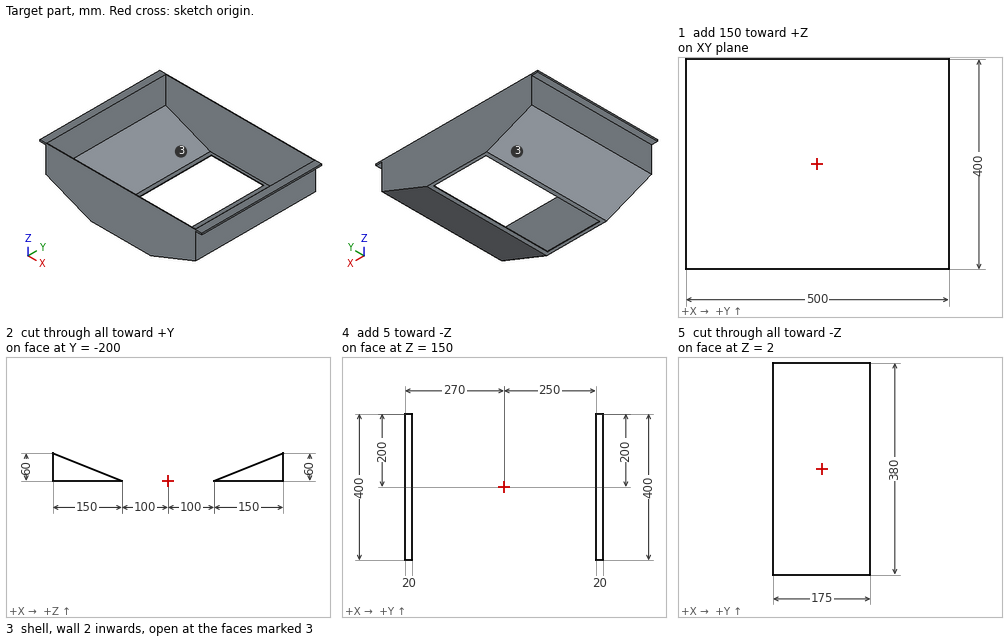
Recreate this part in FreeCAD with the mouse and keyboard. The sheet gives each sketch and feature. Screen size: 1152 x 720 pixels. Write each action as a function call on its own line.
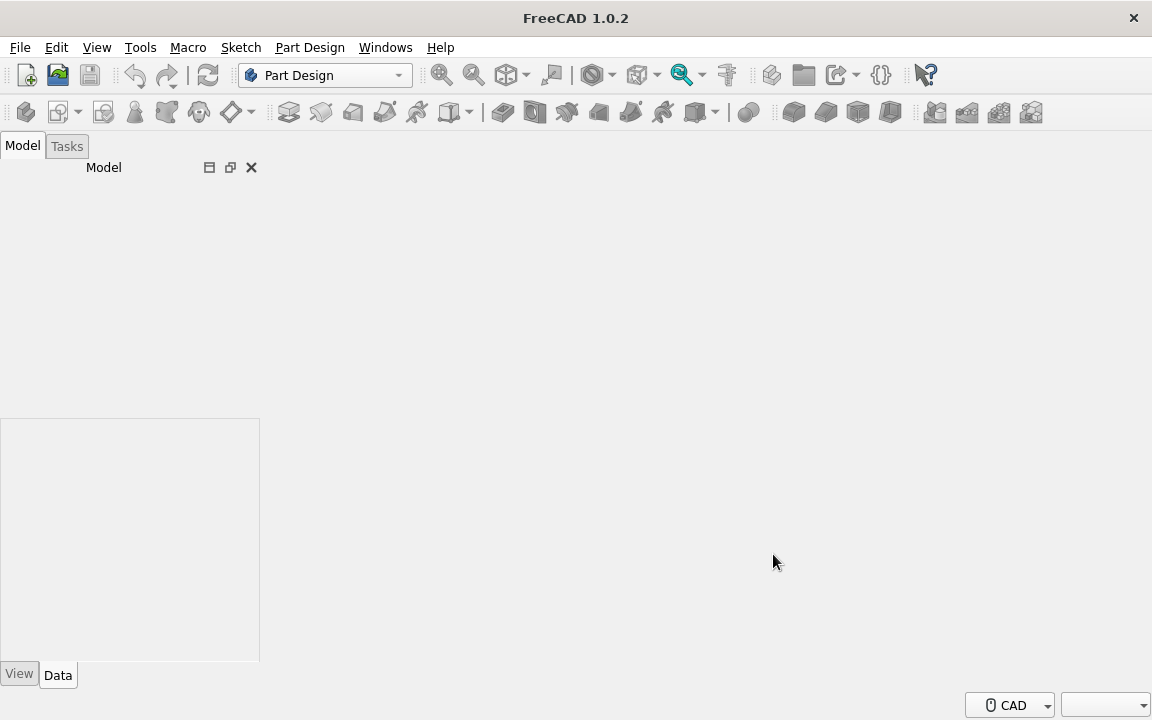
key(ctrl+n)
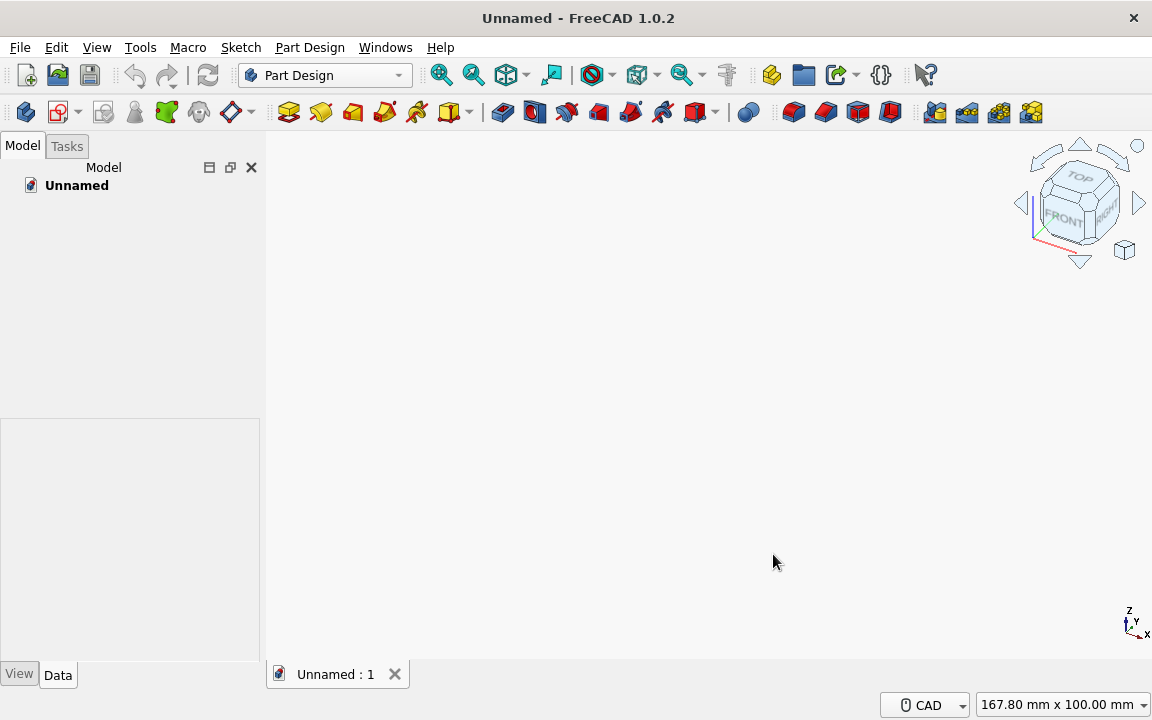
click(58, 112)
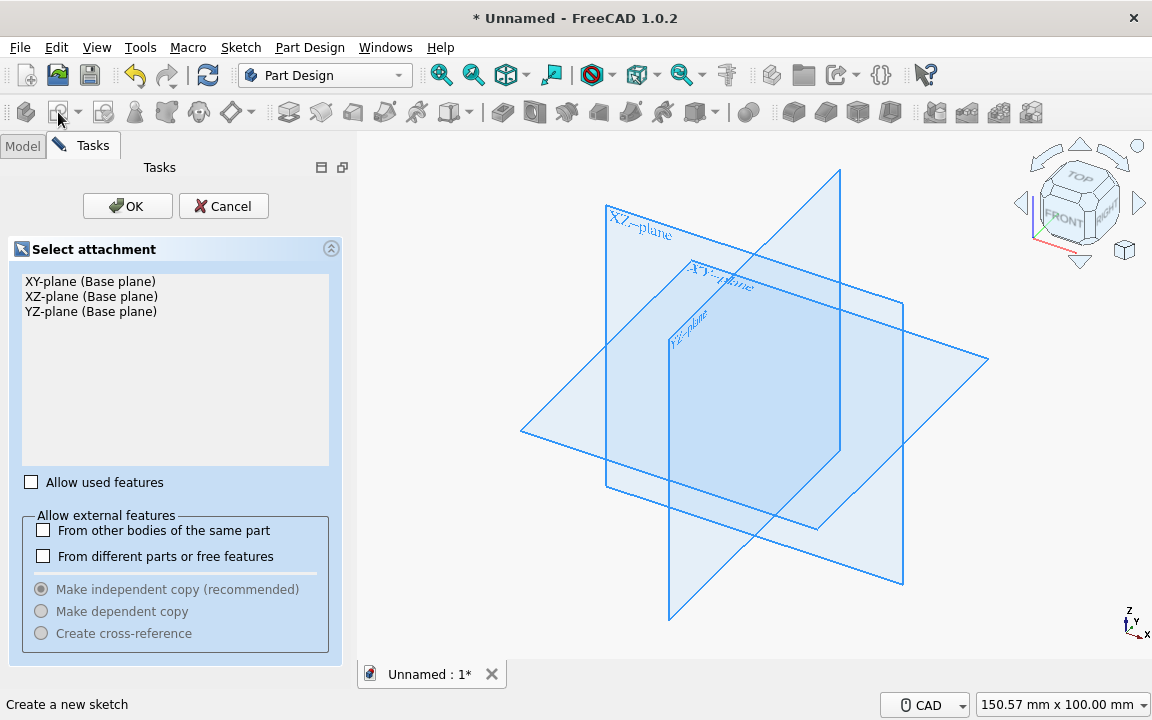
click(82, 282)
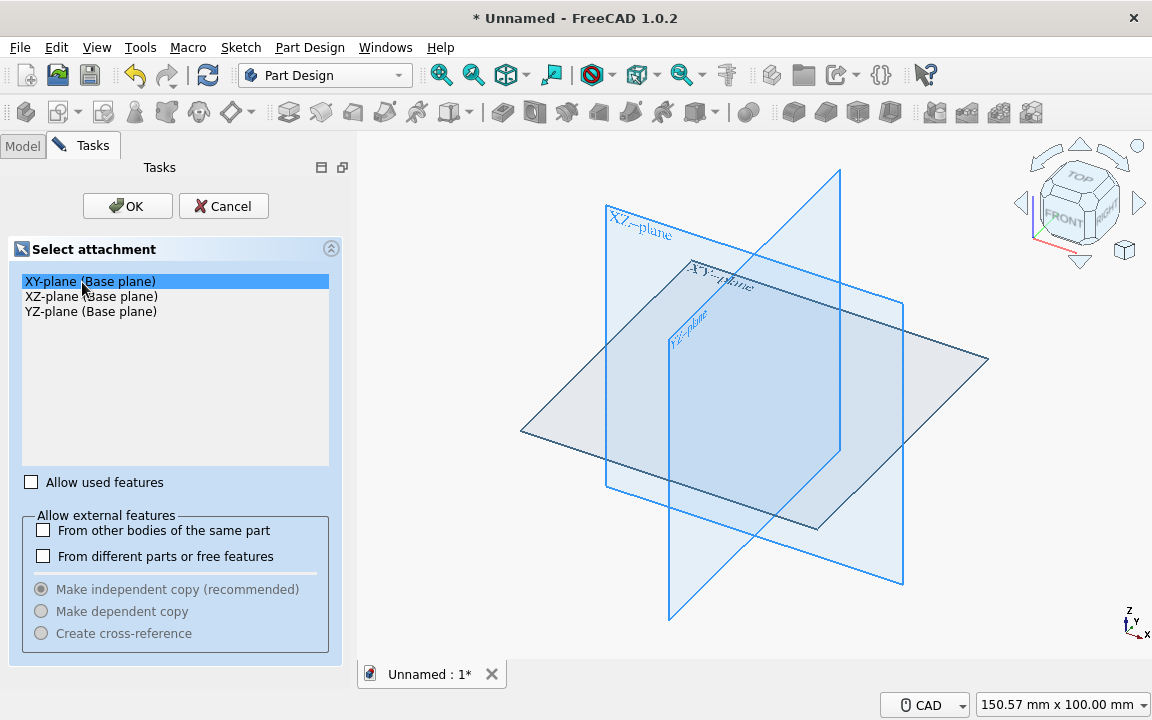
click(128, 206)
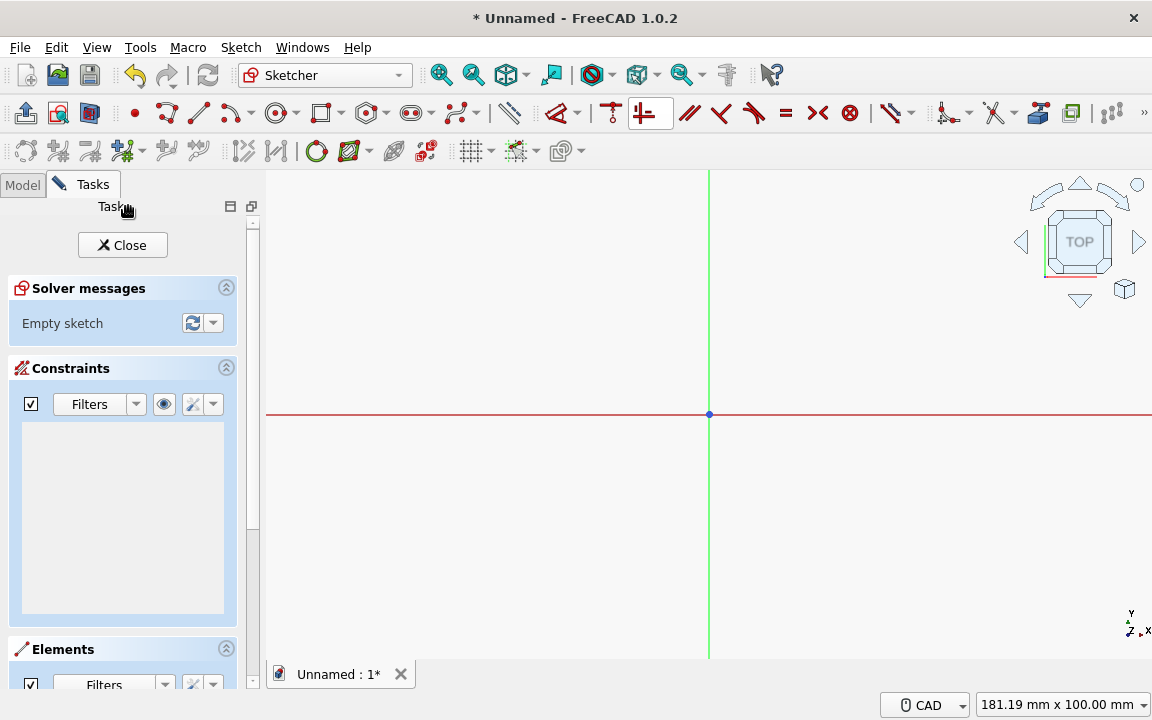
scroll(627, 415, down, 9)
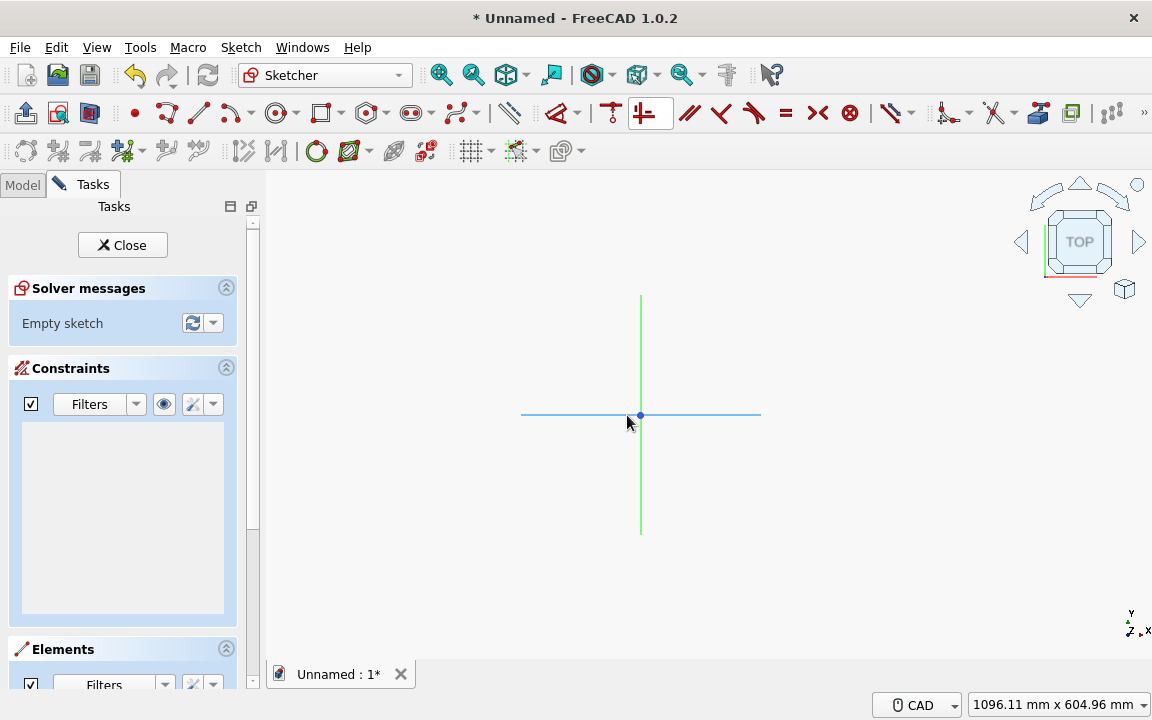
key(g)
key(v)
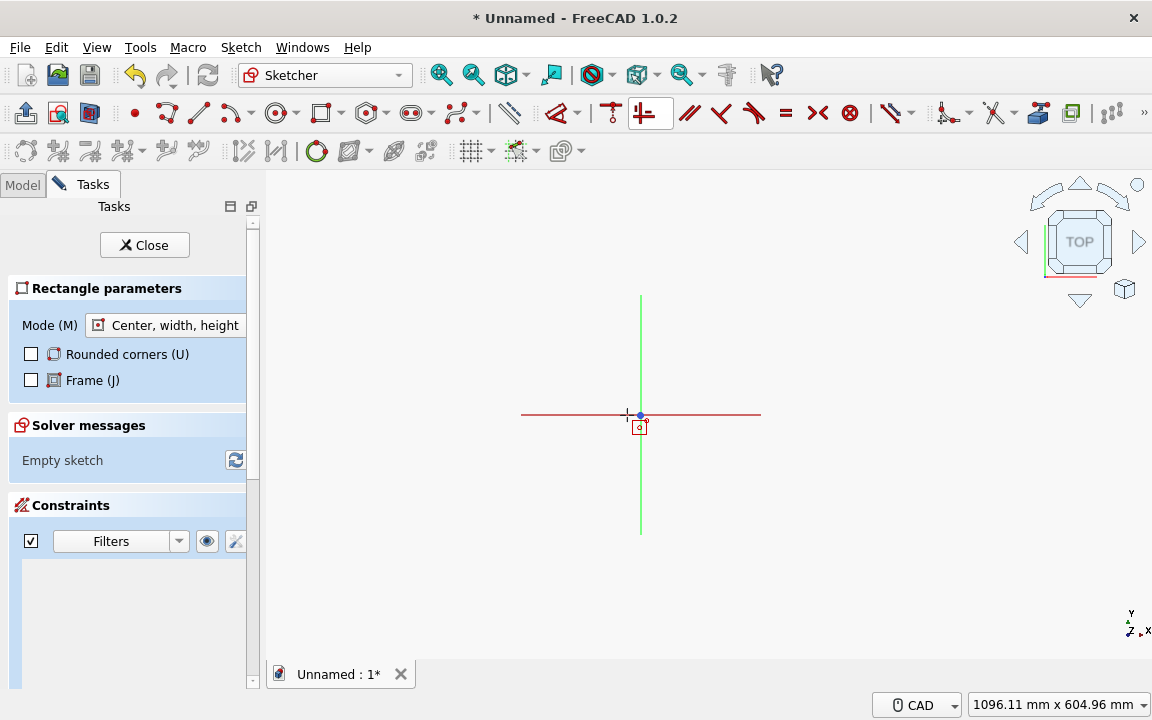
click(641, 415)
click(843, 254)
key(Escape)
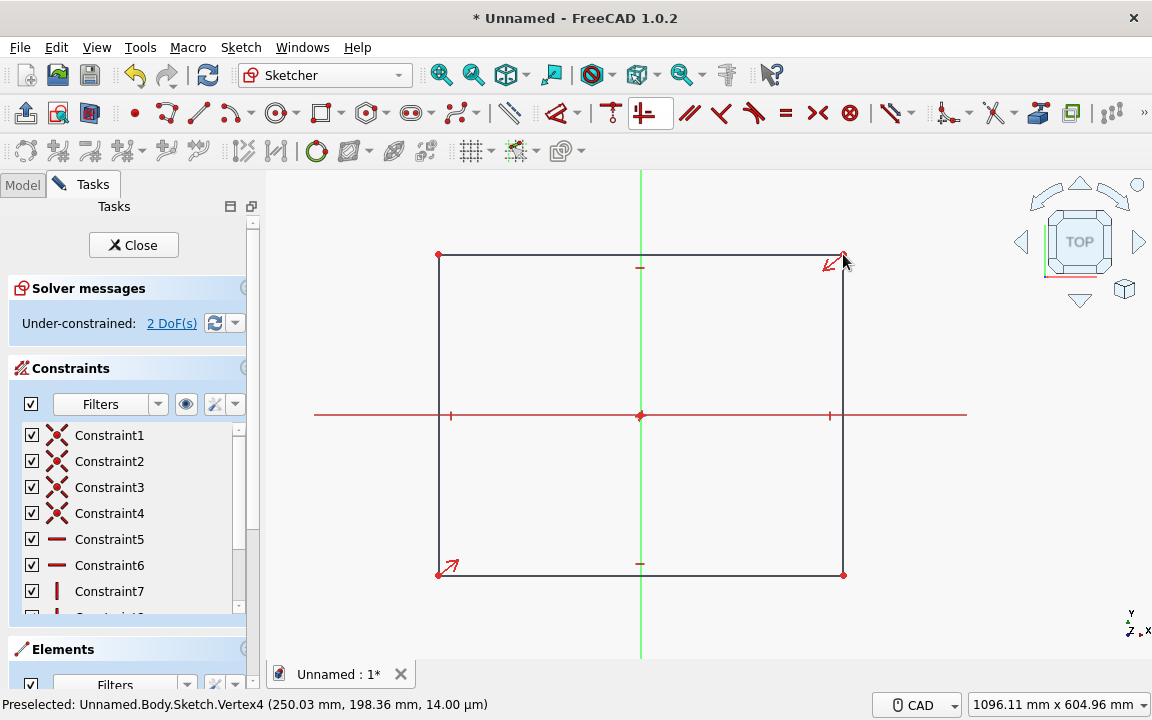
click(560, 576)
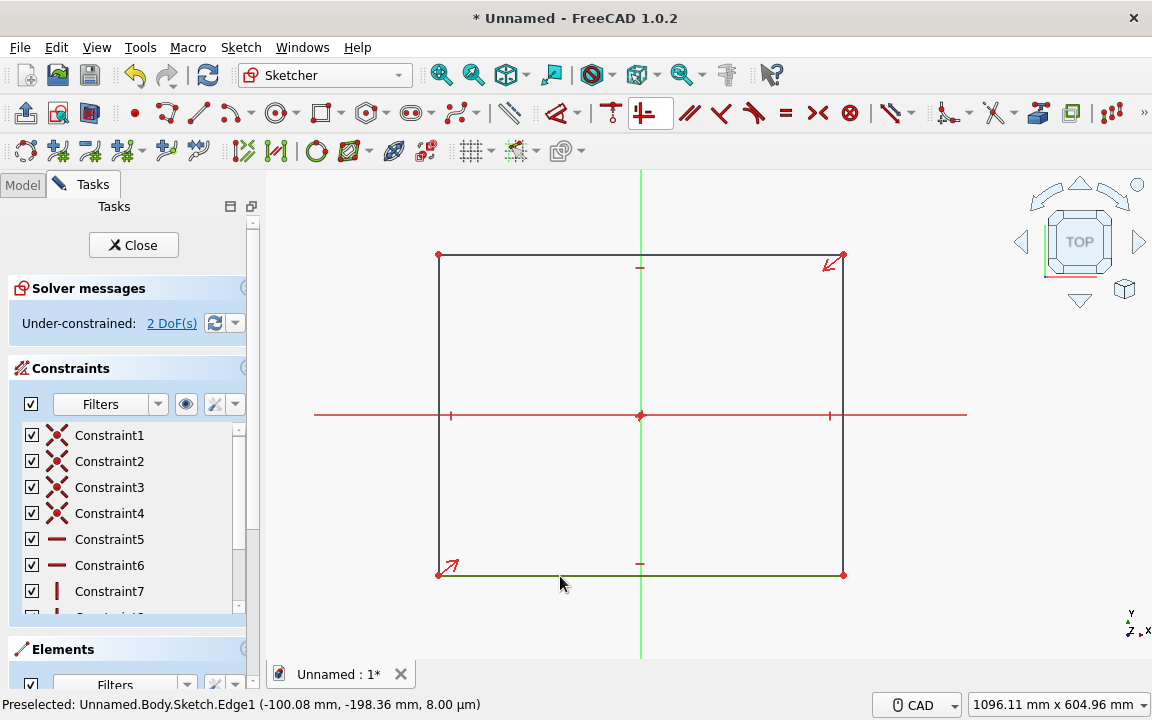
key(l)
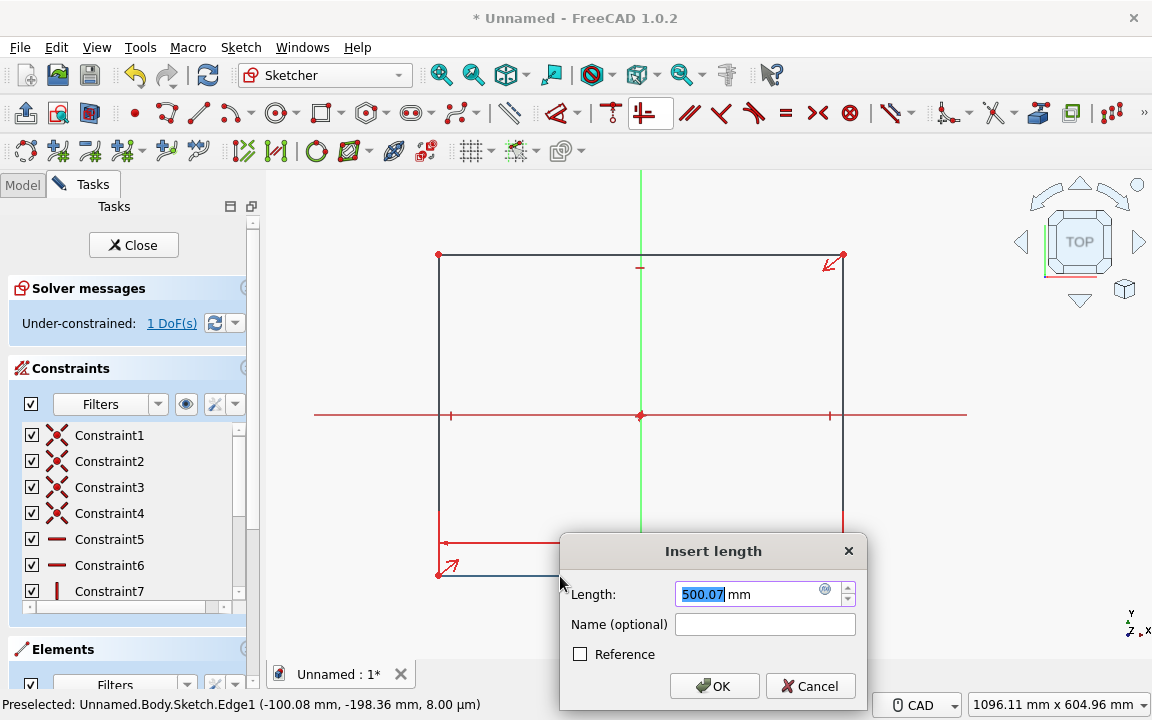
text(500)
key(Return)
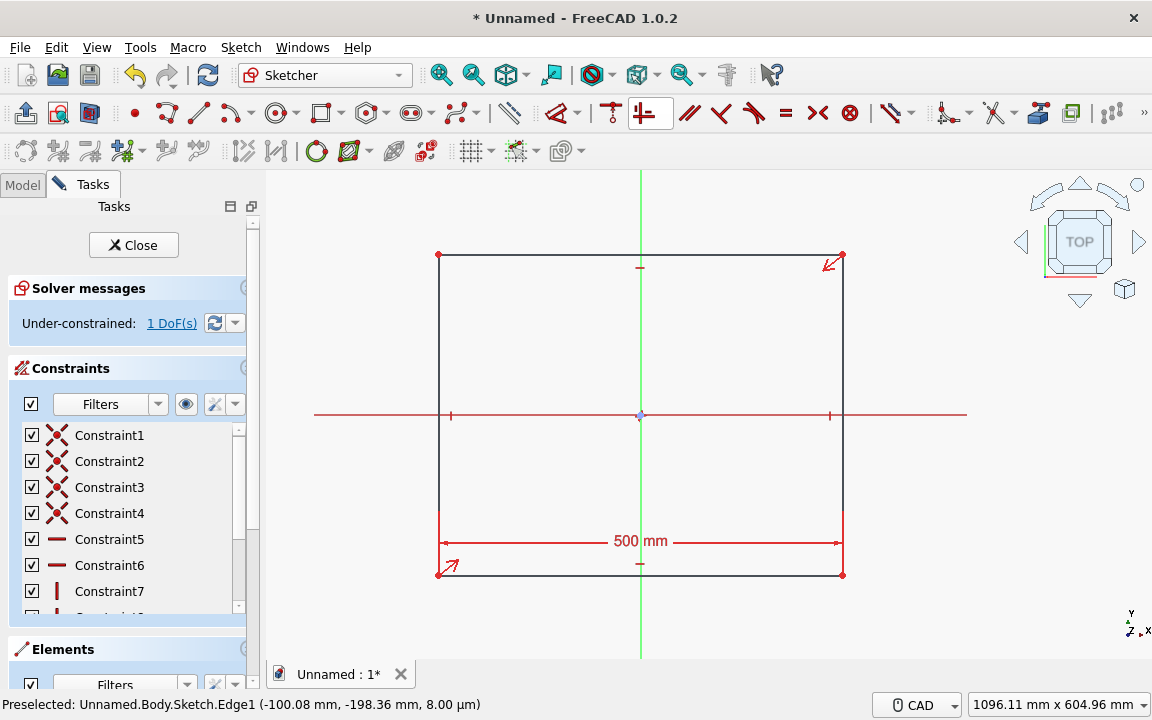
click(843, 479)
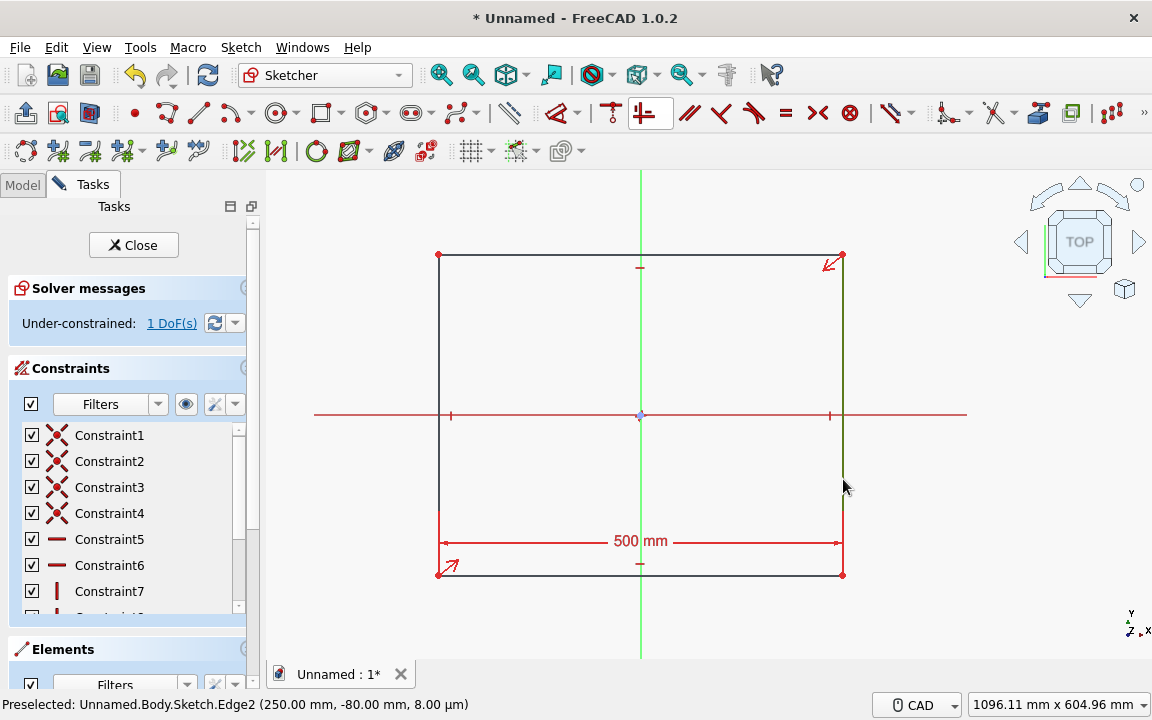
key(i)